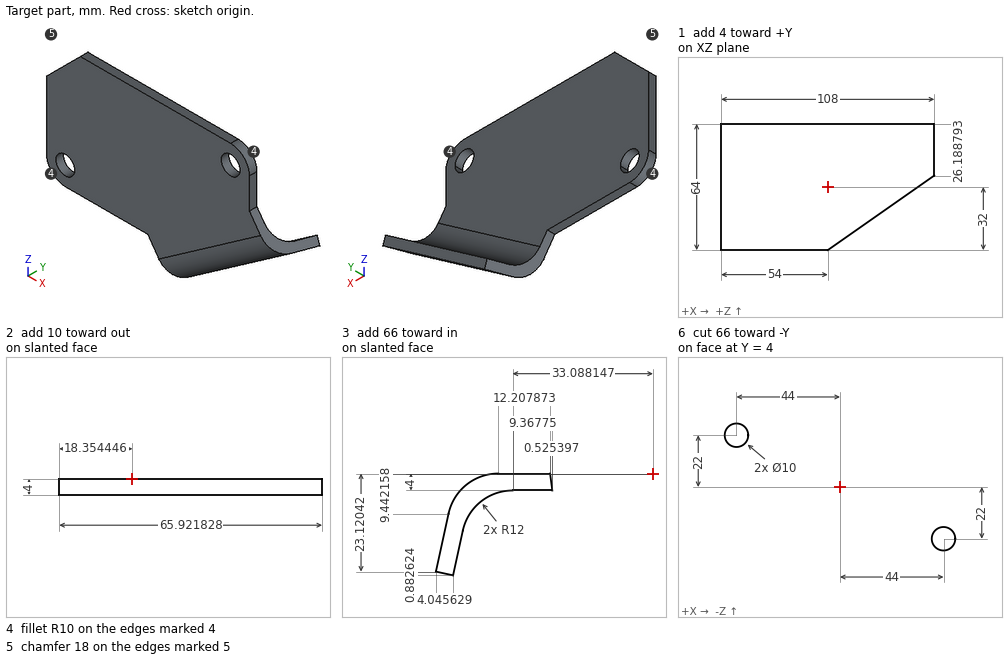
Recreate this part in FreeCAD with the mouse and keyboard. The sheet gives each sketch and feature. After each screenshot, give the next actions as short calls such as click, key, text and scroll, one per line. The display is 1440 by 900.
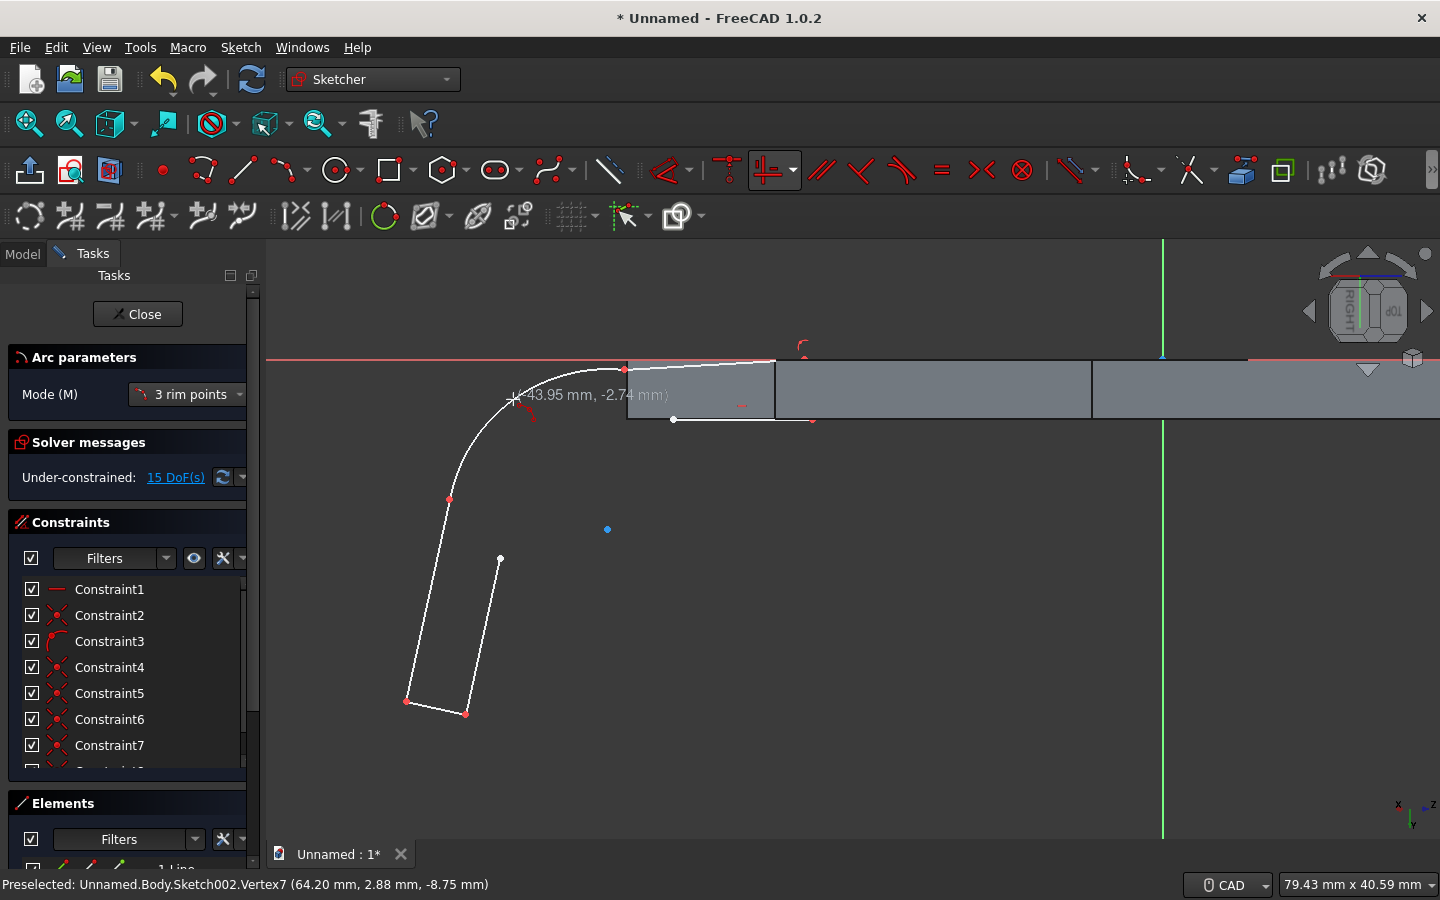
click(500, 559)
click(674, 420)
click(562, 458)
key(Escape)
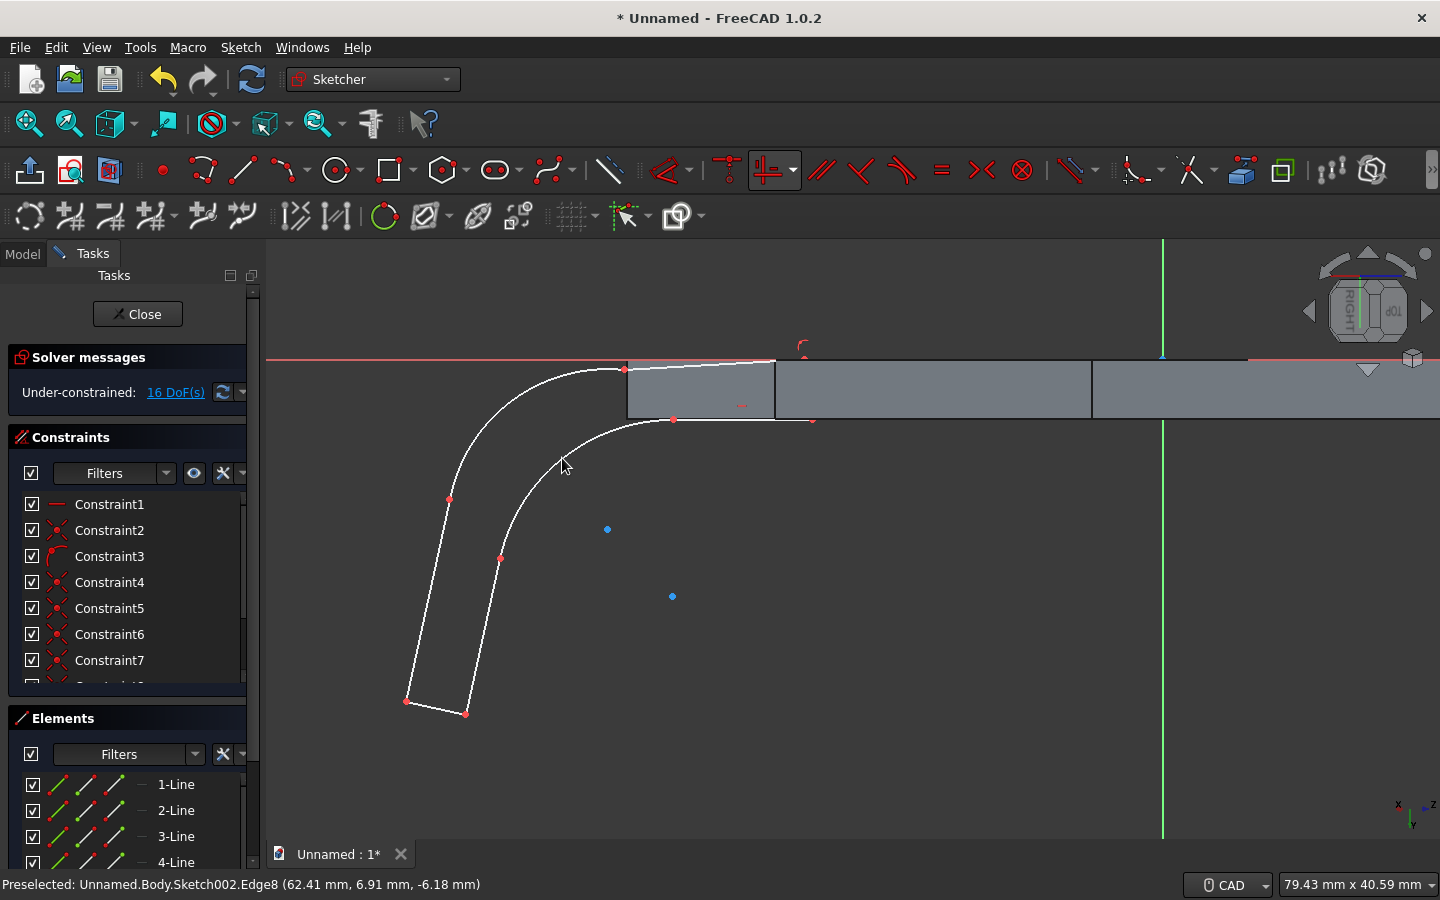
click(715, 420)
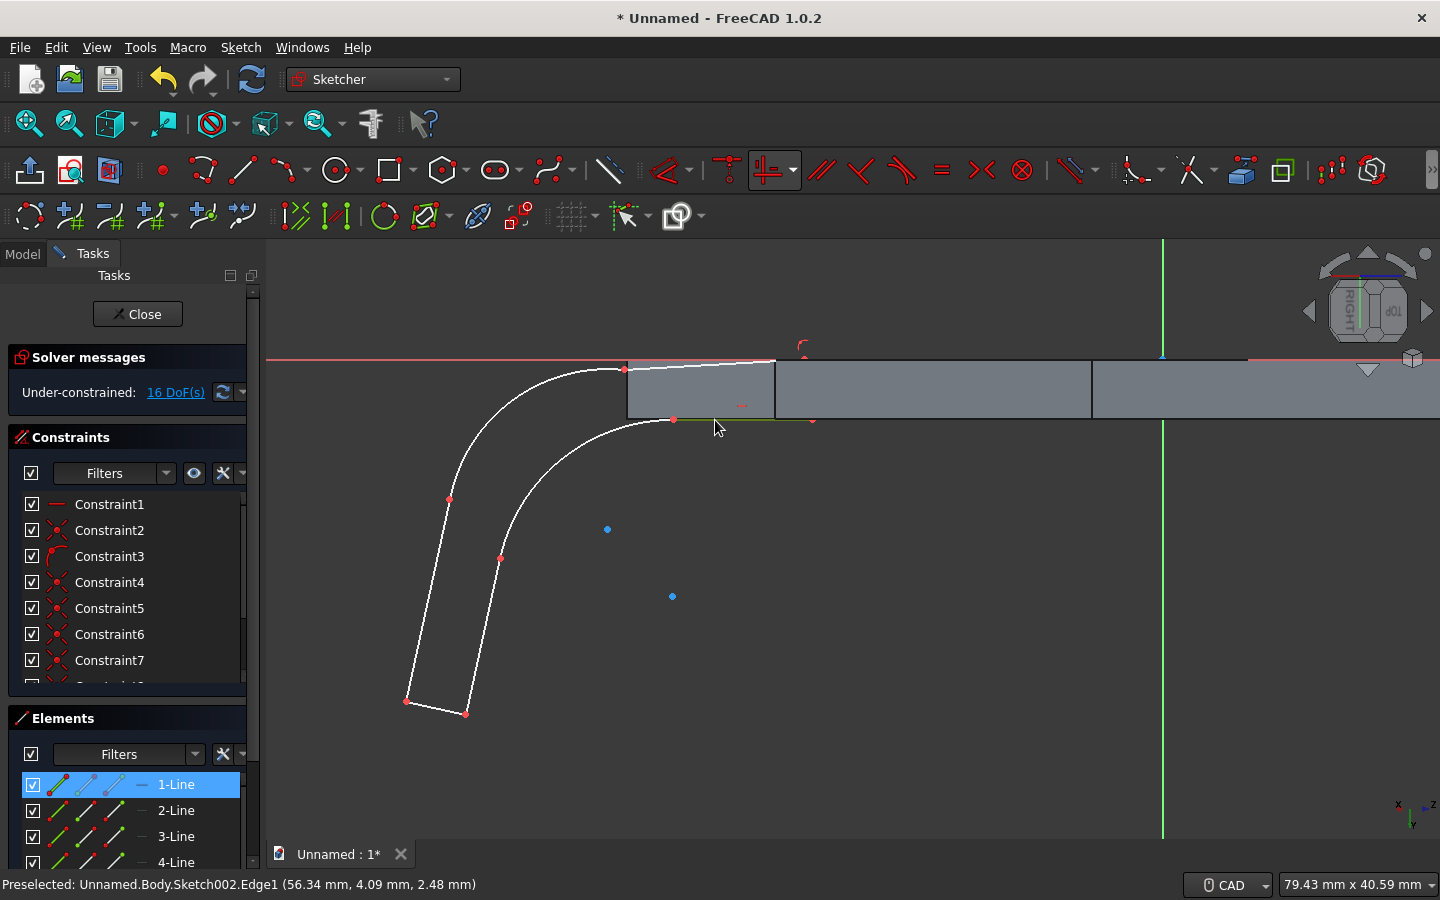
click(604, 434)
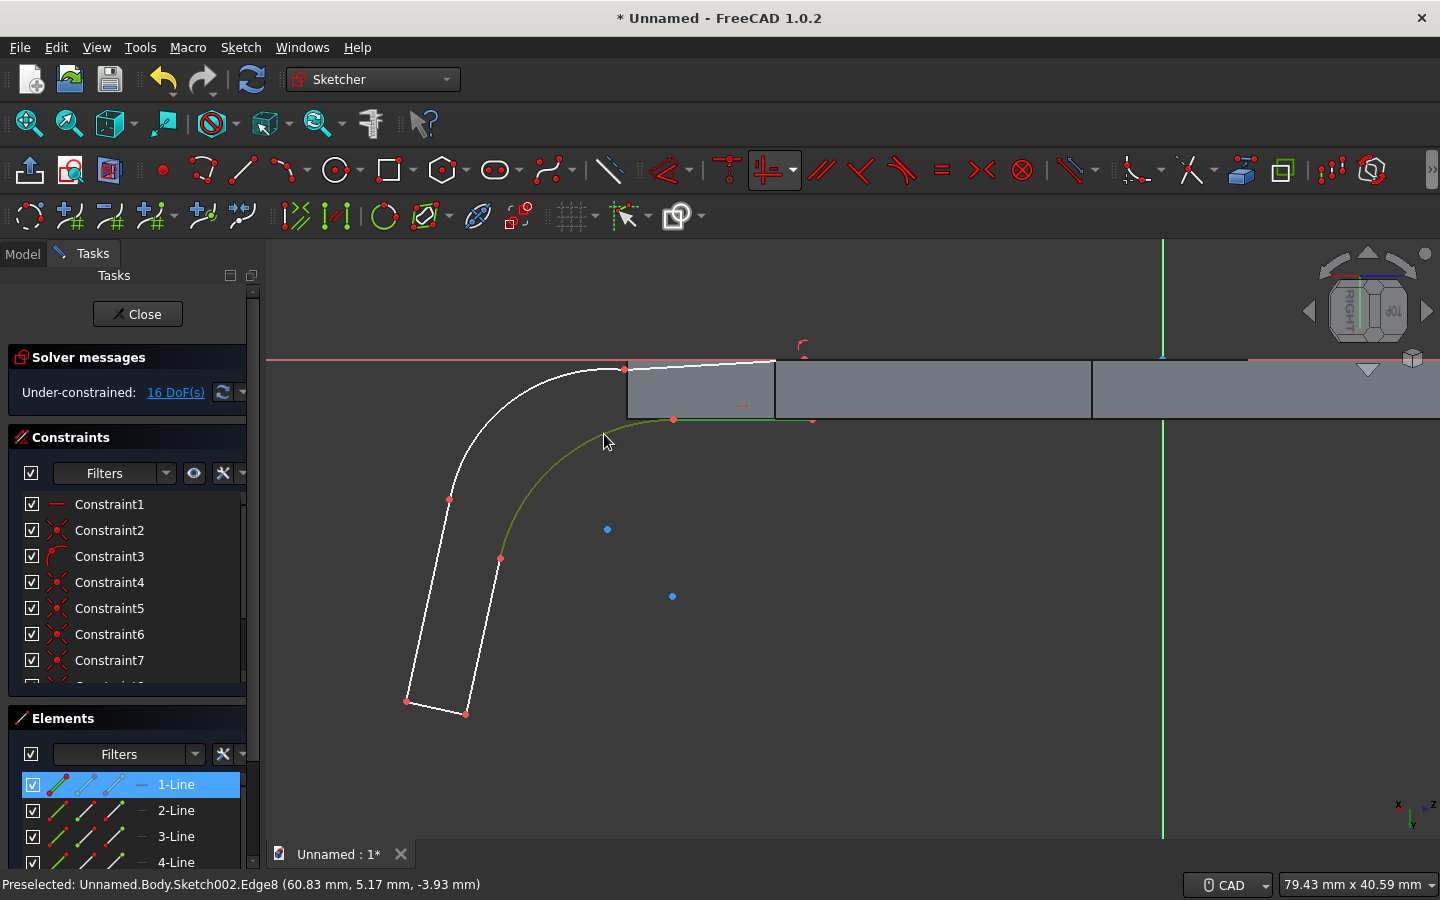
key(t)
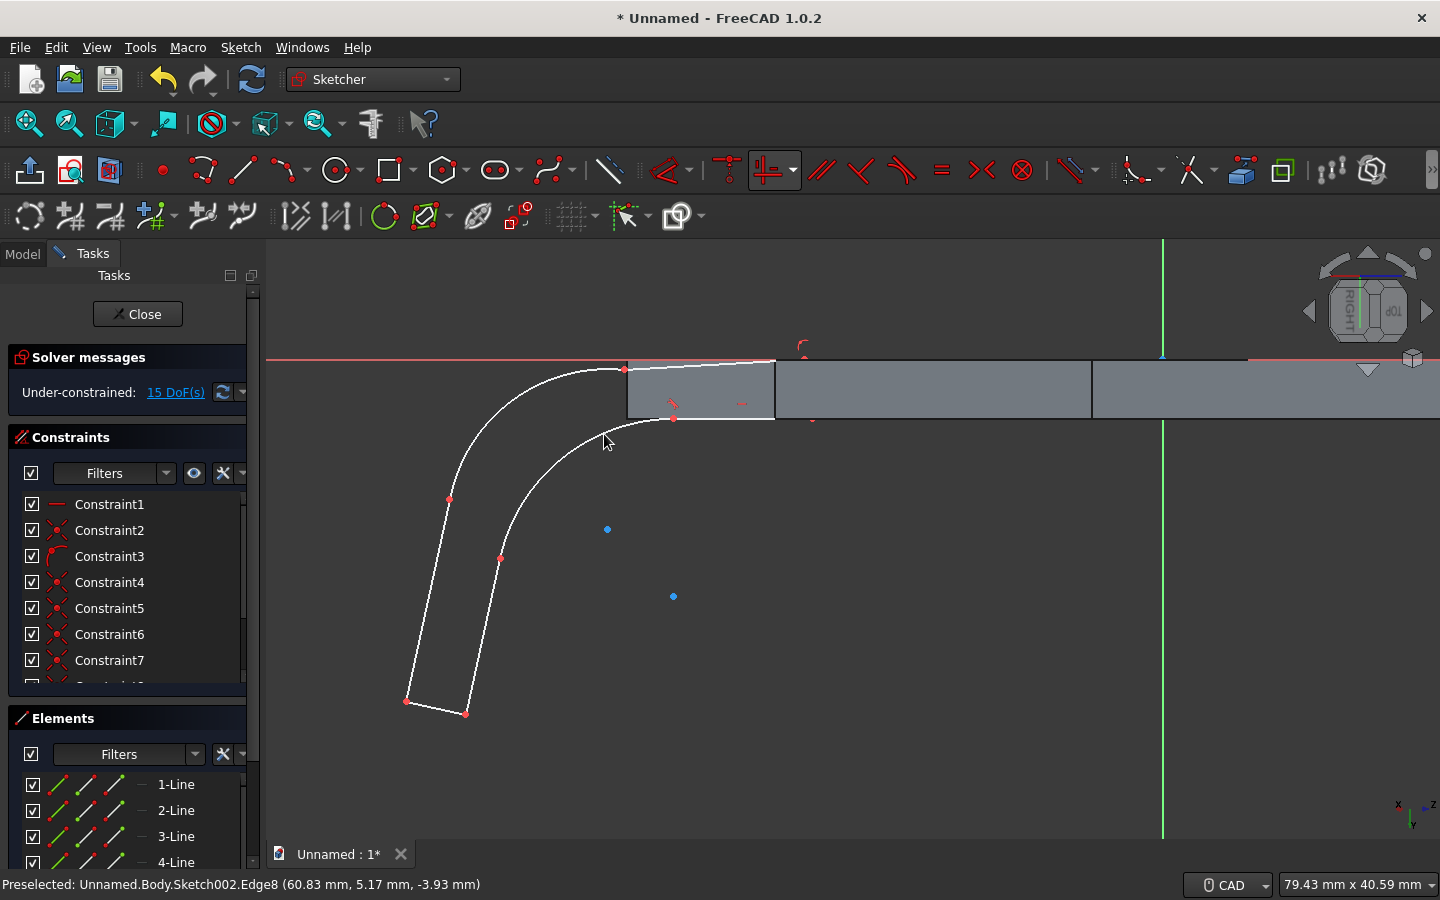
click(750, 363)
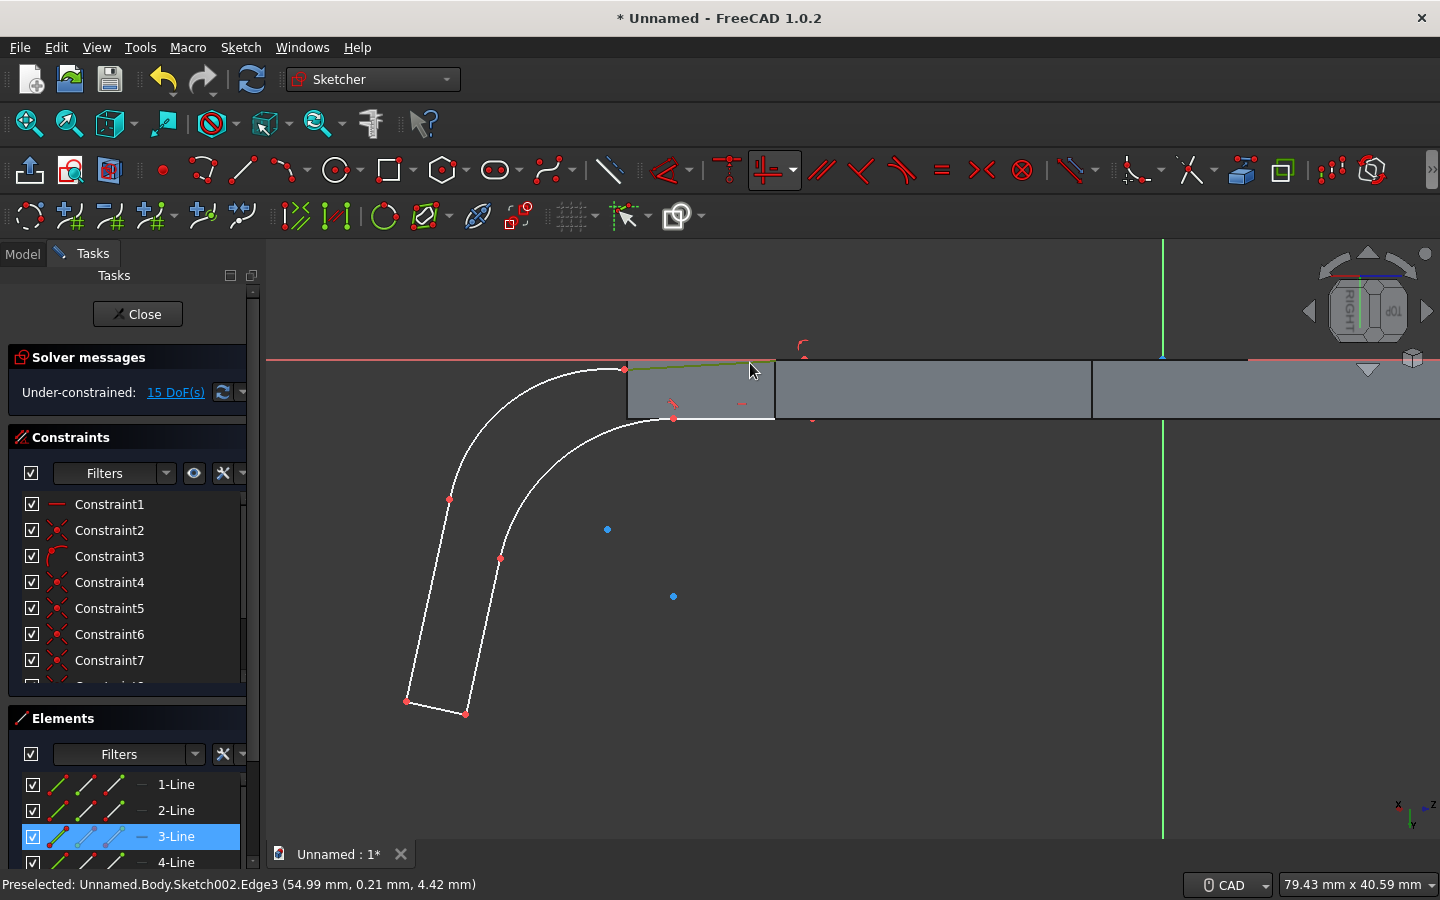
click(554, 379)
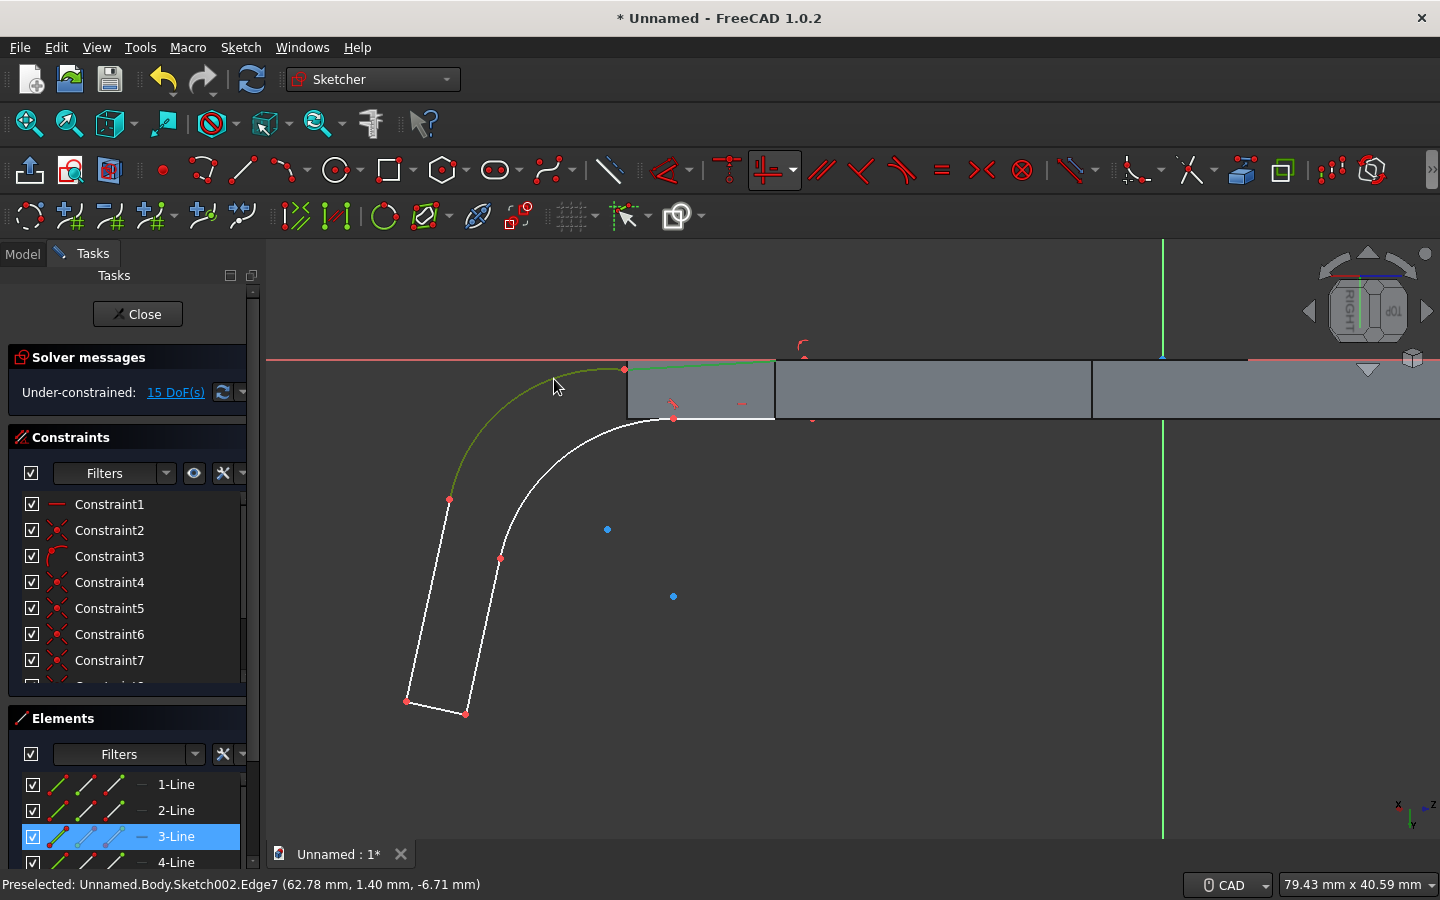
key(t)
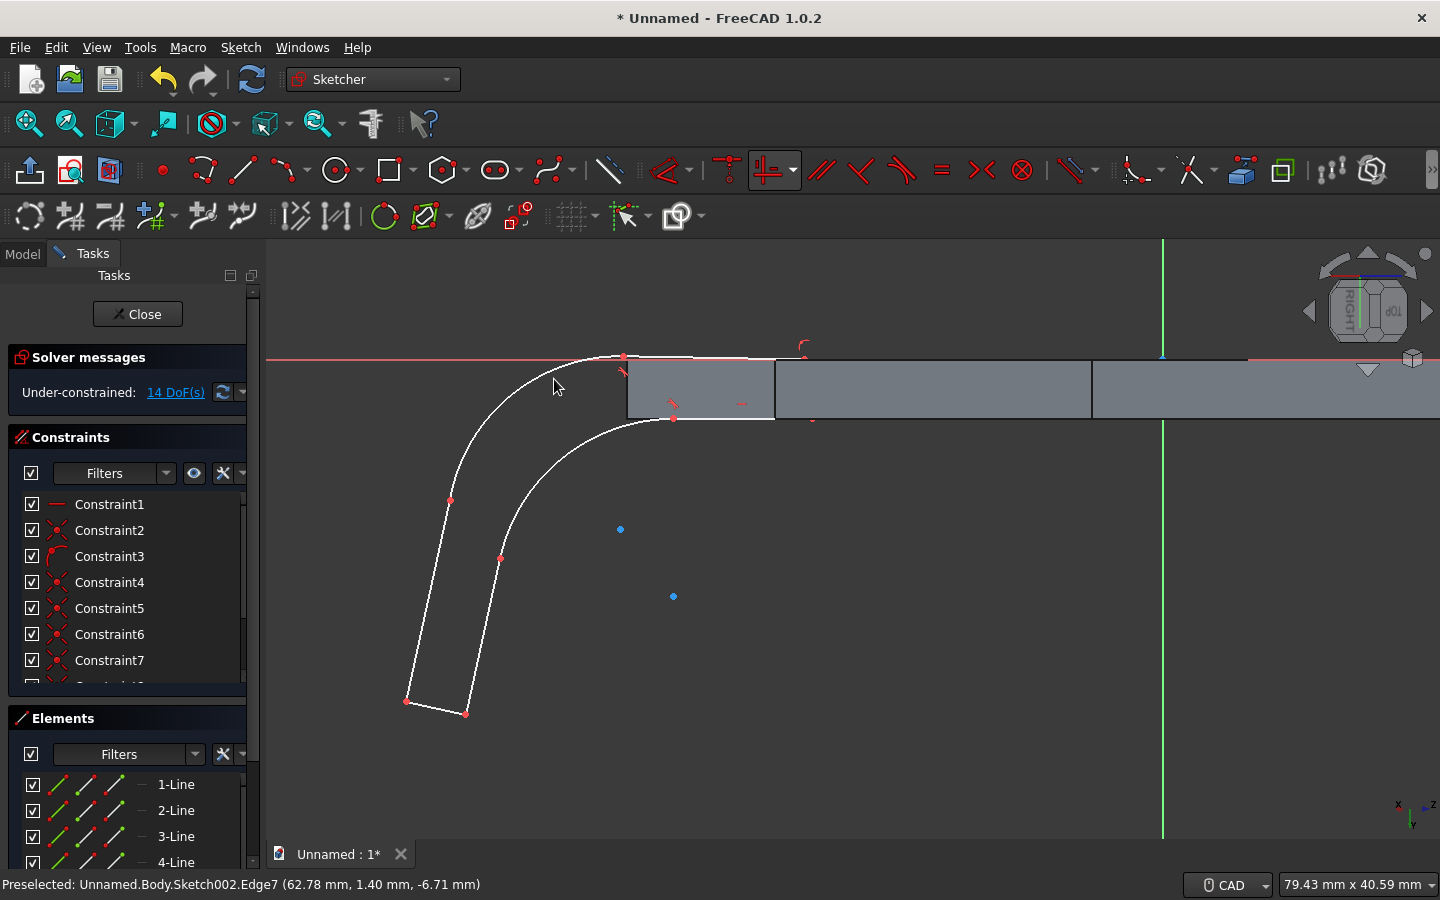
click(437, 561)